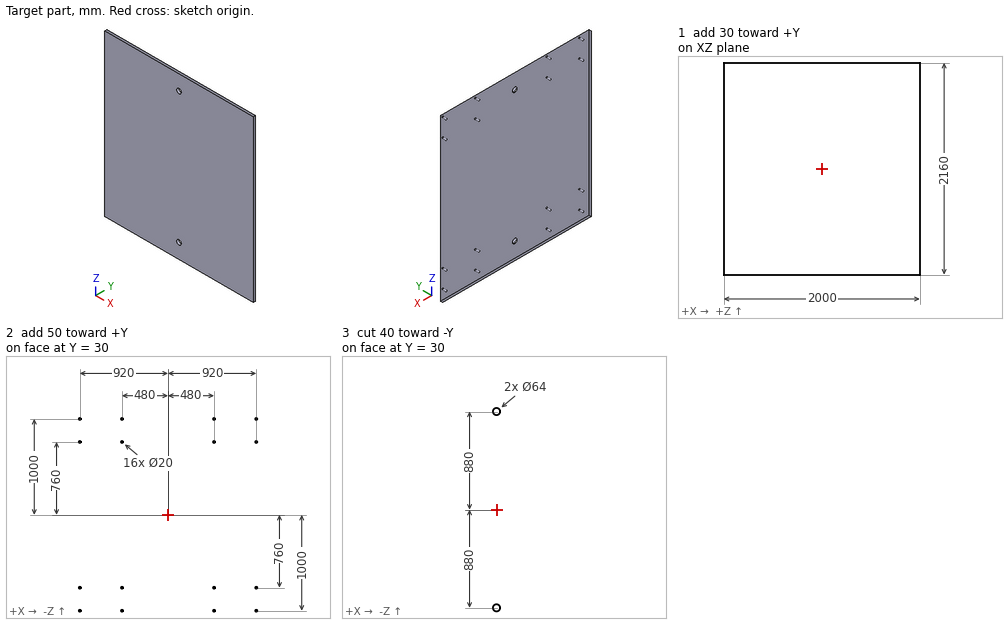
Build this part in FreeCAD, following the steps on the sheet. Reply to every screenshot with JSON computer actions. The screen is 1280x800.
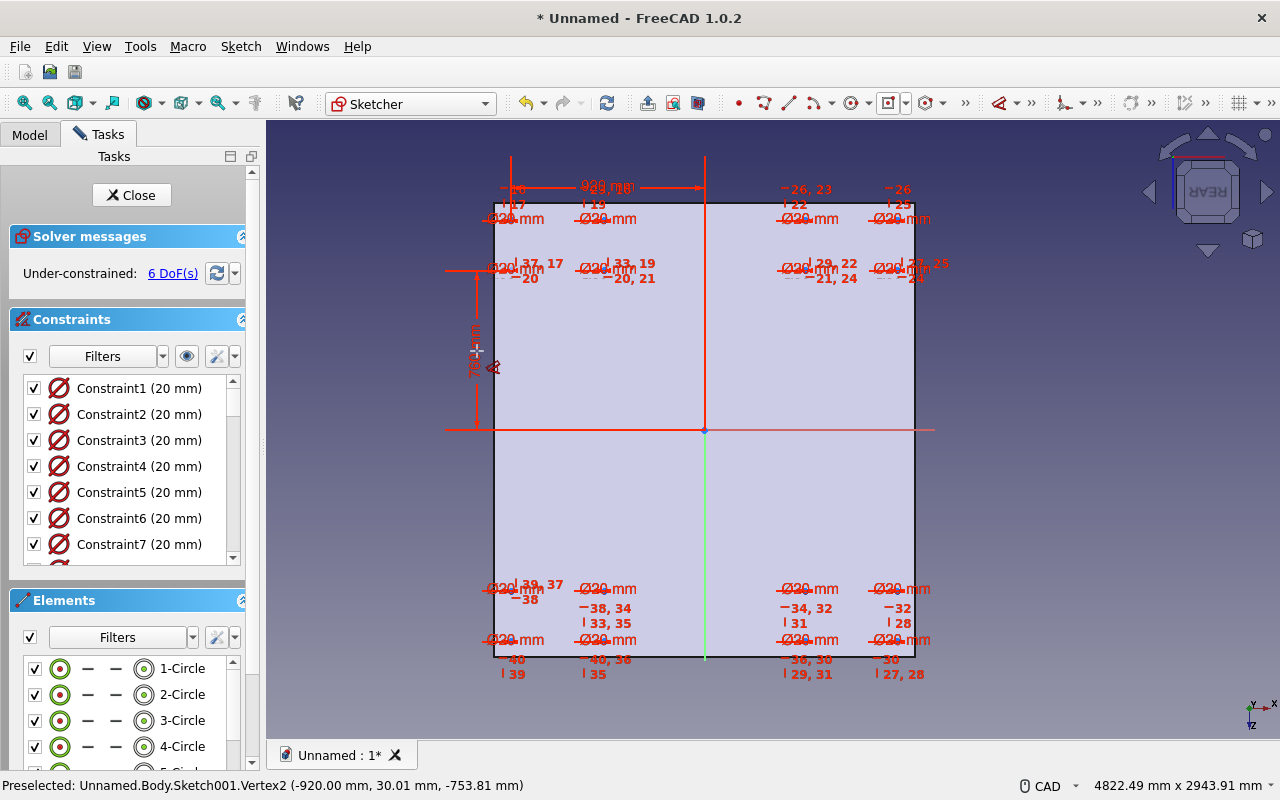
{"action": "left_click", "coordinate": [604, 221]}
{"action": "left_click", "coordinate": [690, 187]}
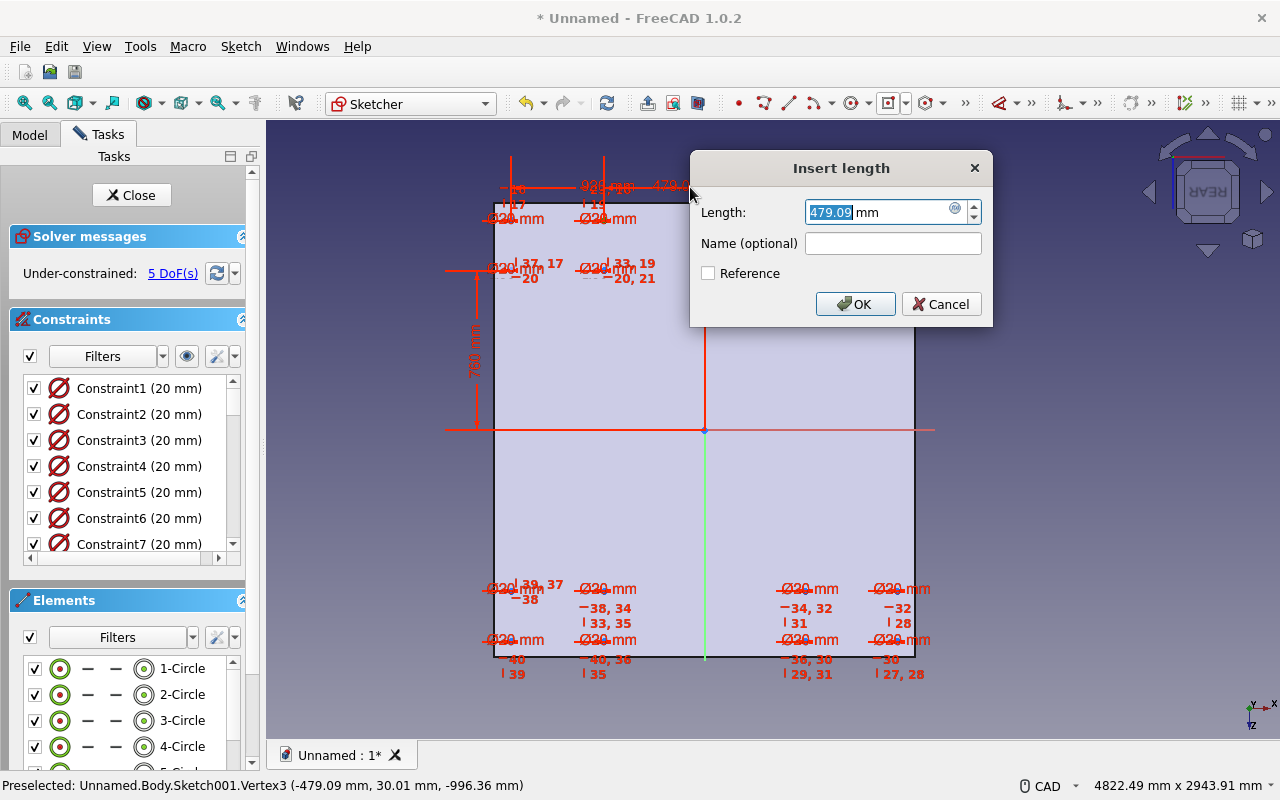
{"action": "type", "text": "480"}
{"action": "key", "text": "Return"}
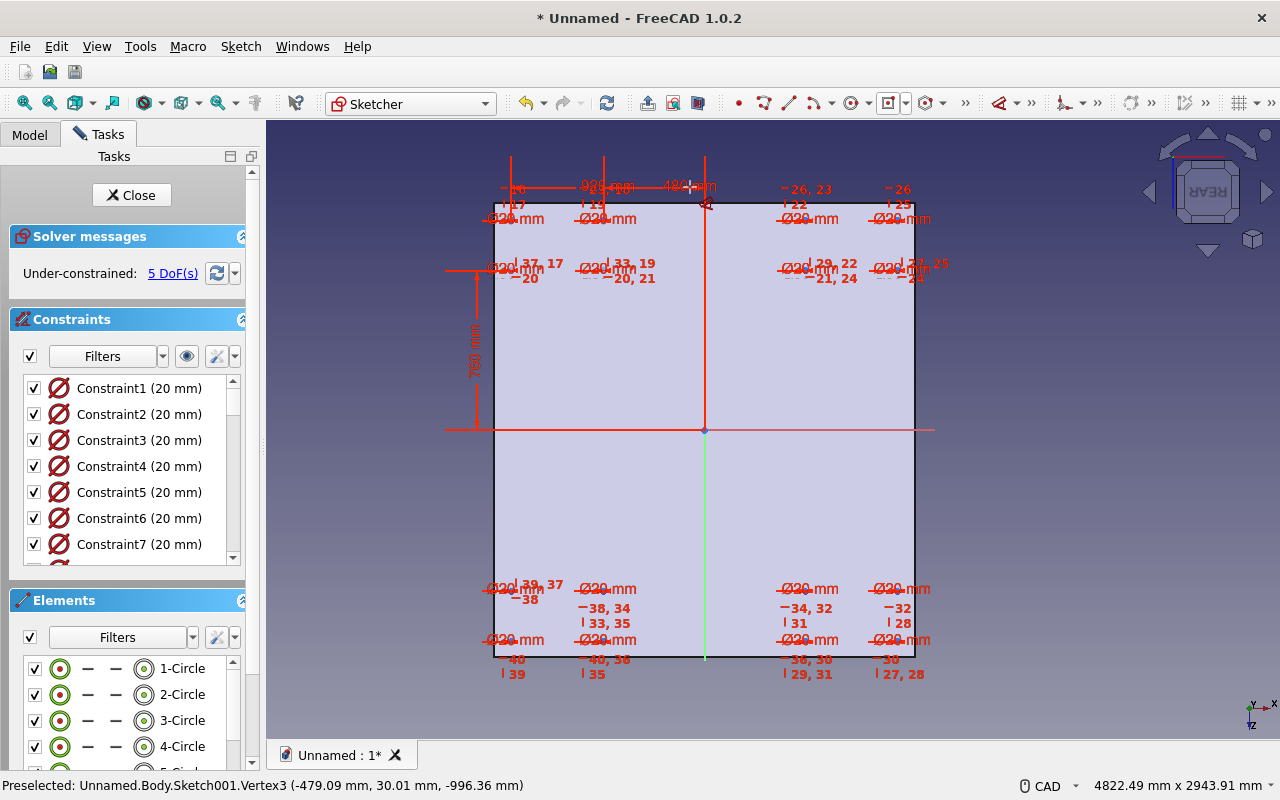
{"action": "left_click", "coordinate": [806, 271]}
{"action": "left_click", "coordinate": [755, 237]}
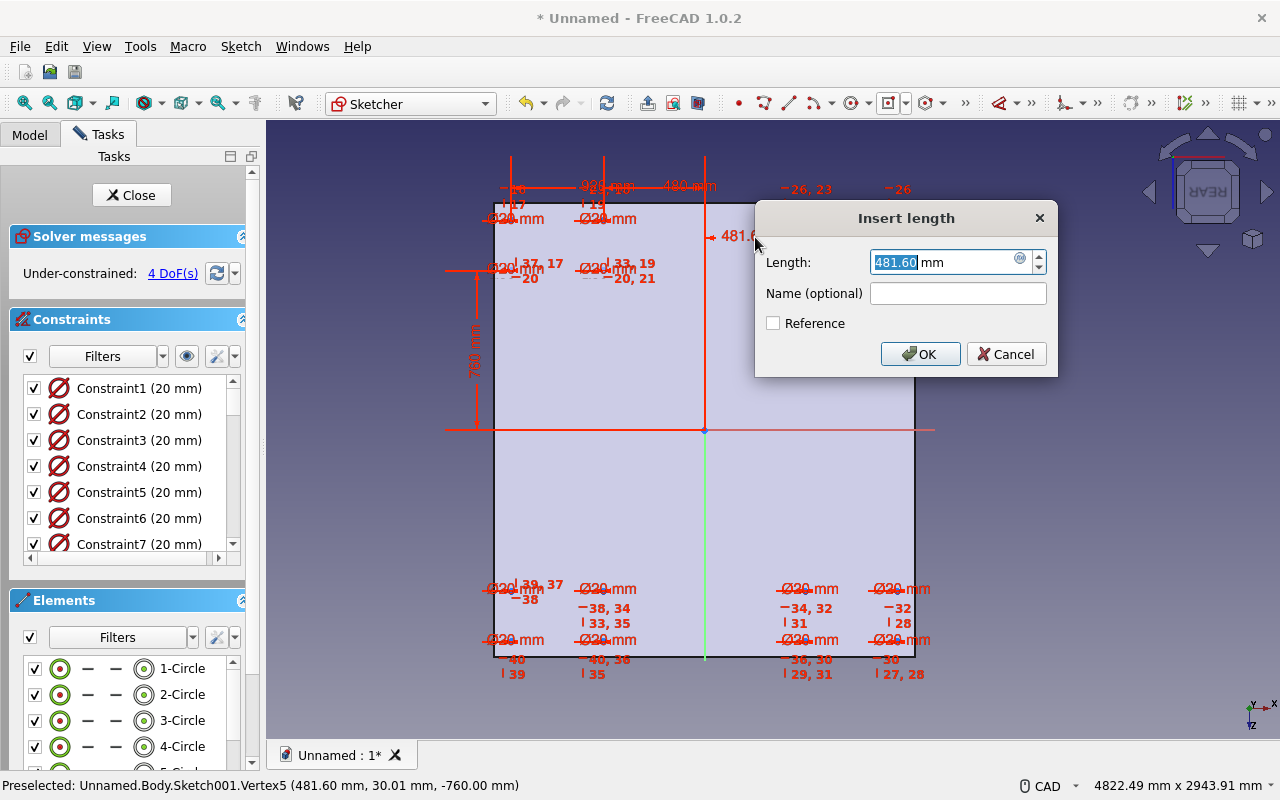
{"action": "type", "text": "480"}
{"action": "key", "text": "Return"}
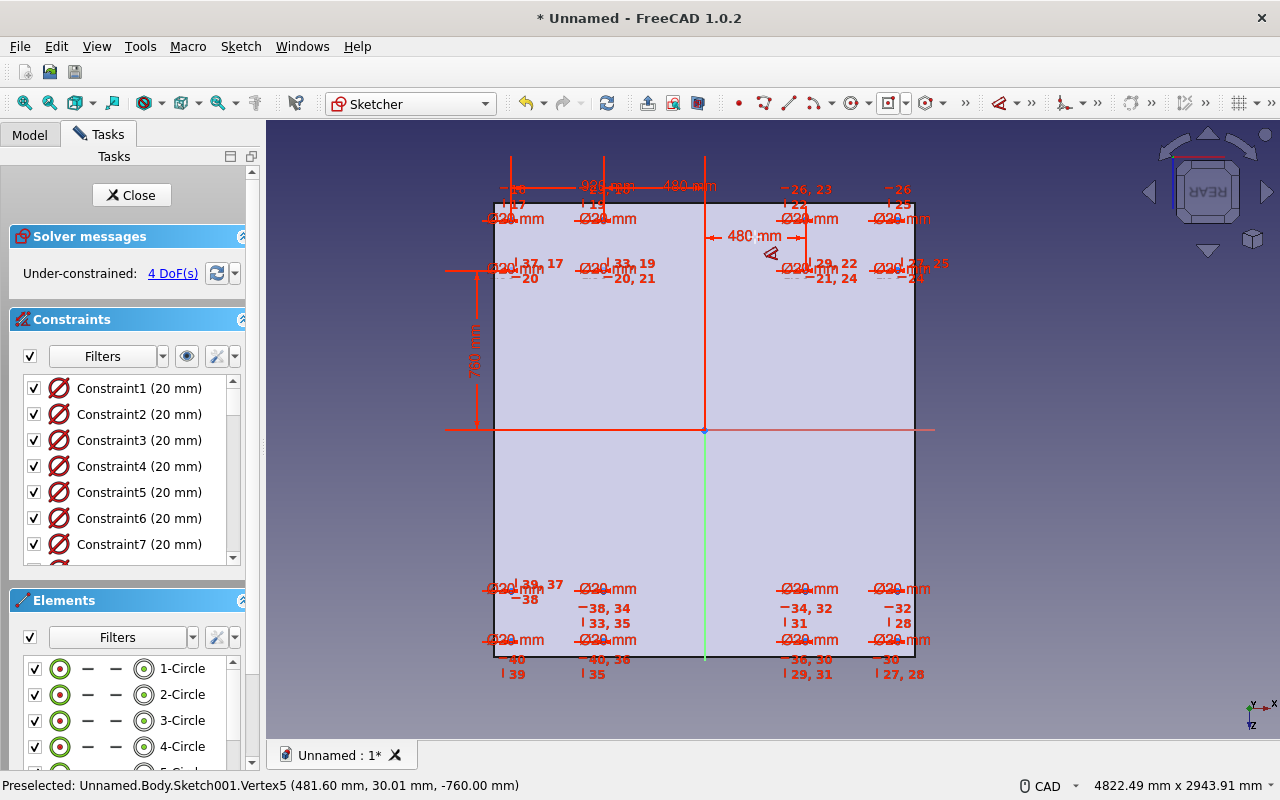
{"action": "left_click", "coordinate": [898, 271]}
{"action": "left_click", "coordinate": [846, 237]}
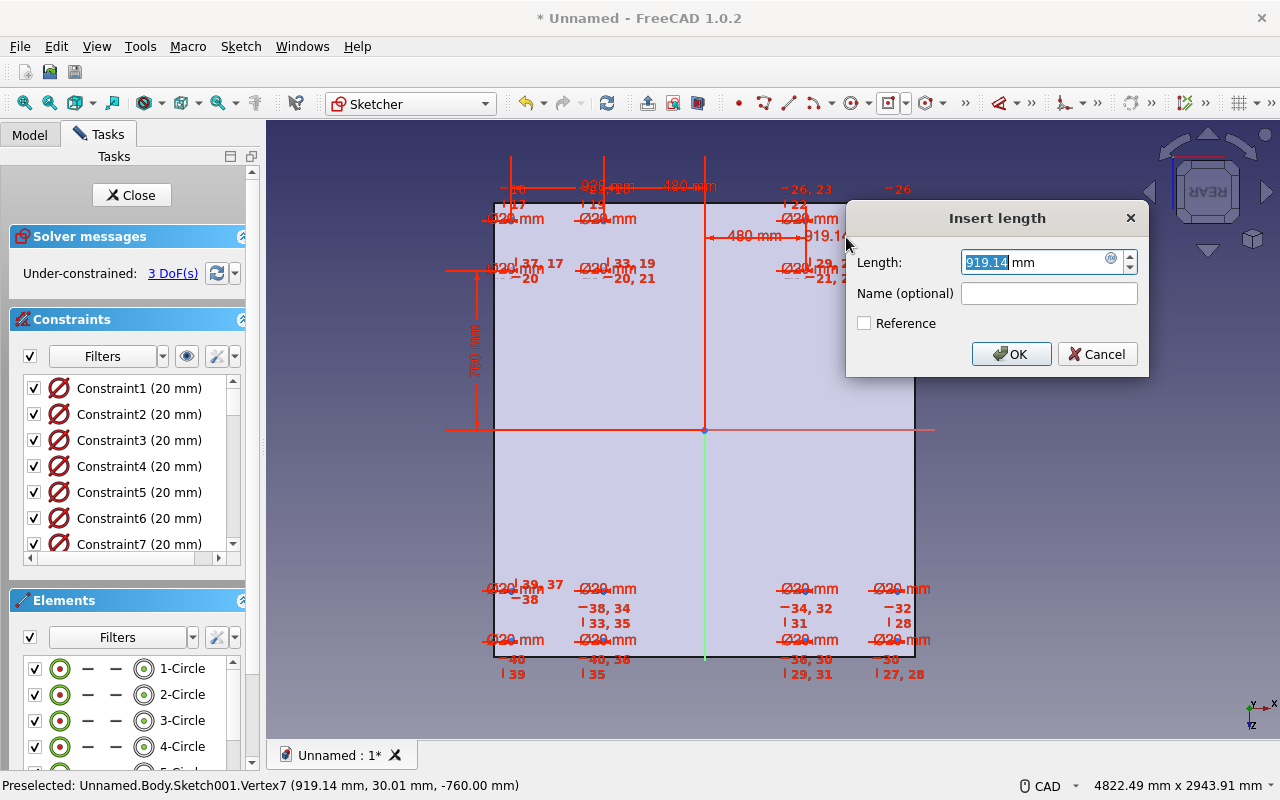
{"action": "type", "text": "920"}
{"action": "key", "text": "Return"}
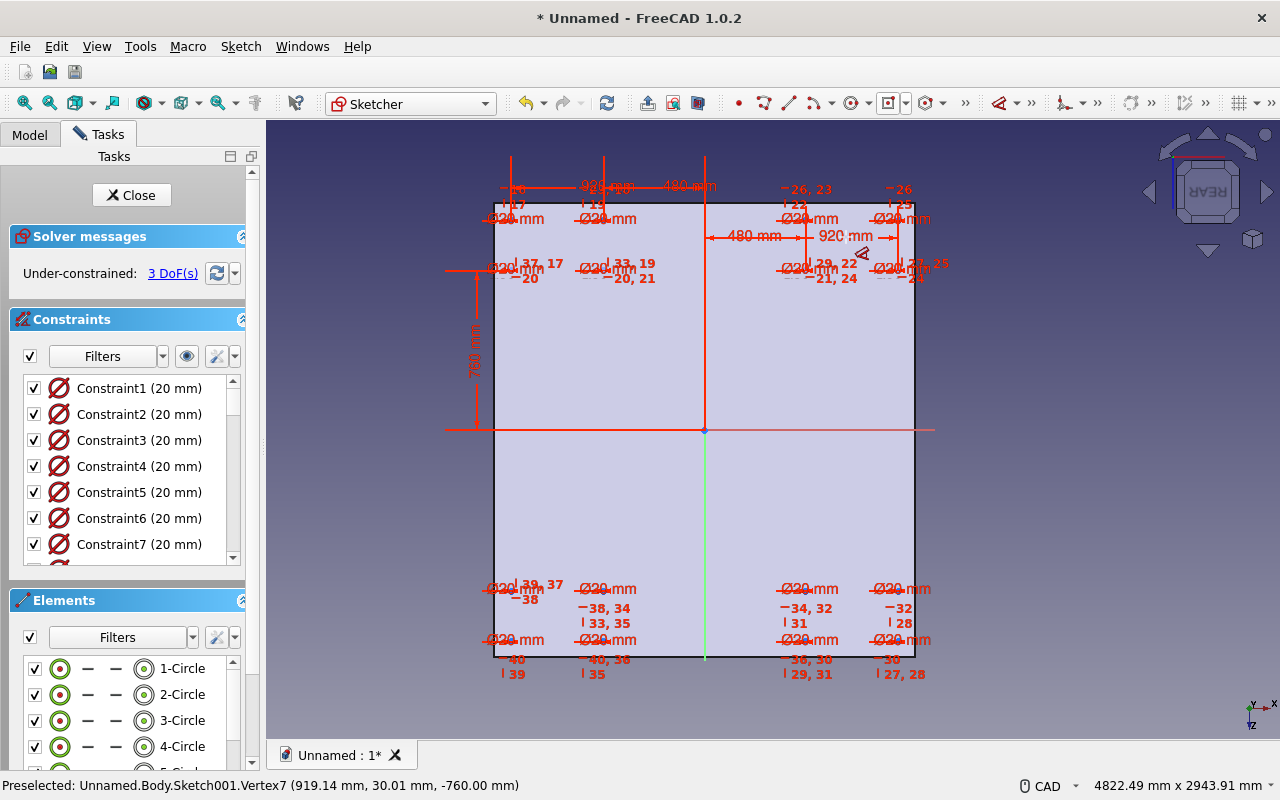
{"action": "left_click", "coordinate": [898, 591]}
{"action": "left_click", "coordinate": [932, 511]}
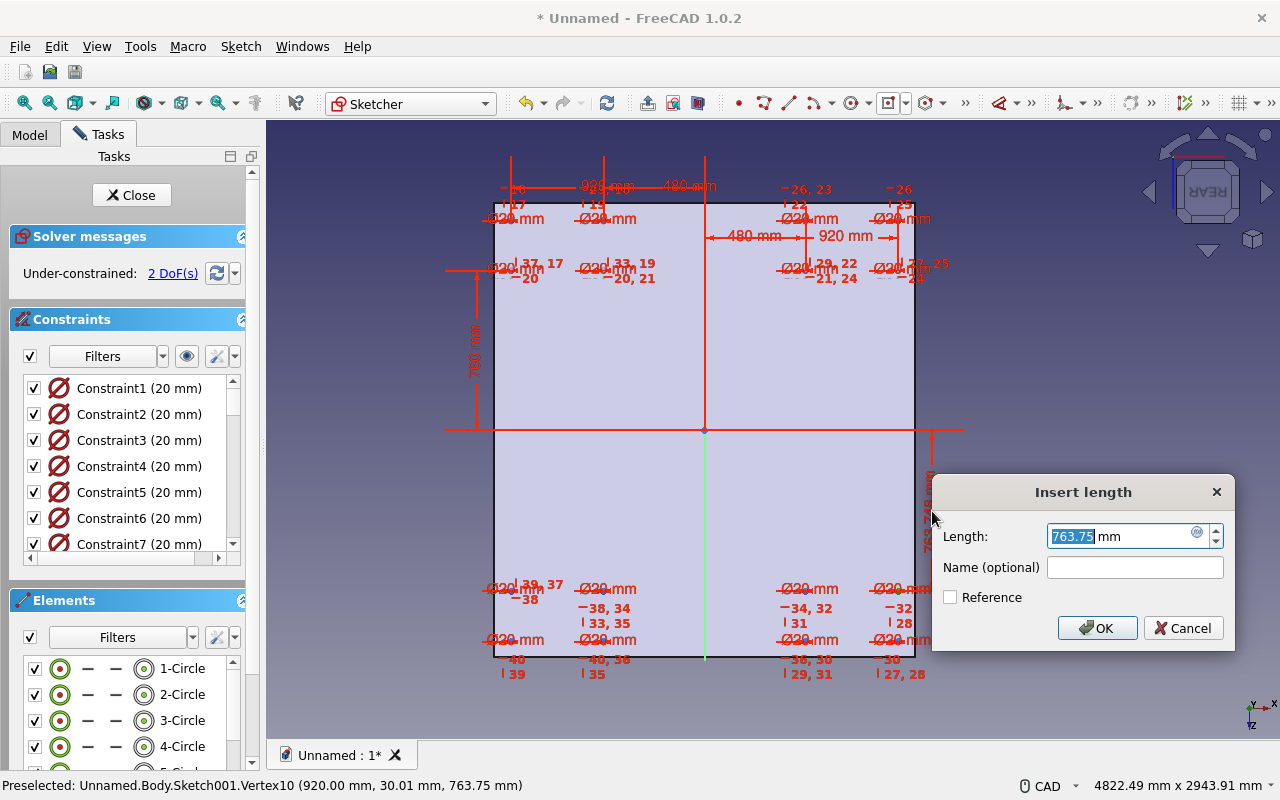
{"action": "type", "text": "760"}
{"action": "key", "text": "Return"}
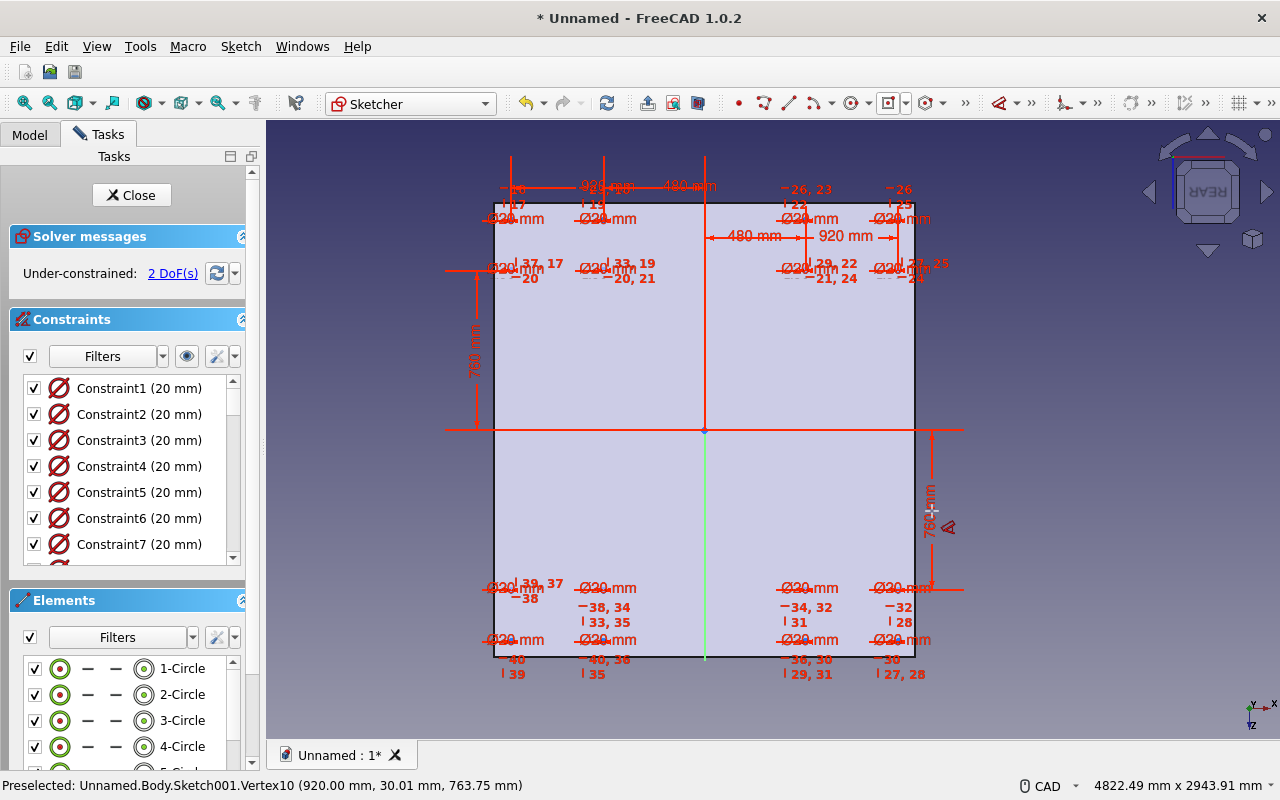
{"action": "left_click", "coordinate": [511, 221]}
{"action": "left_click", "coordinate": [477, 326]}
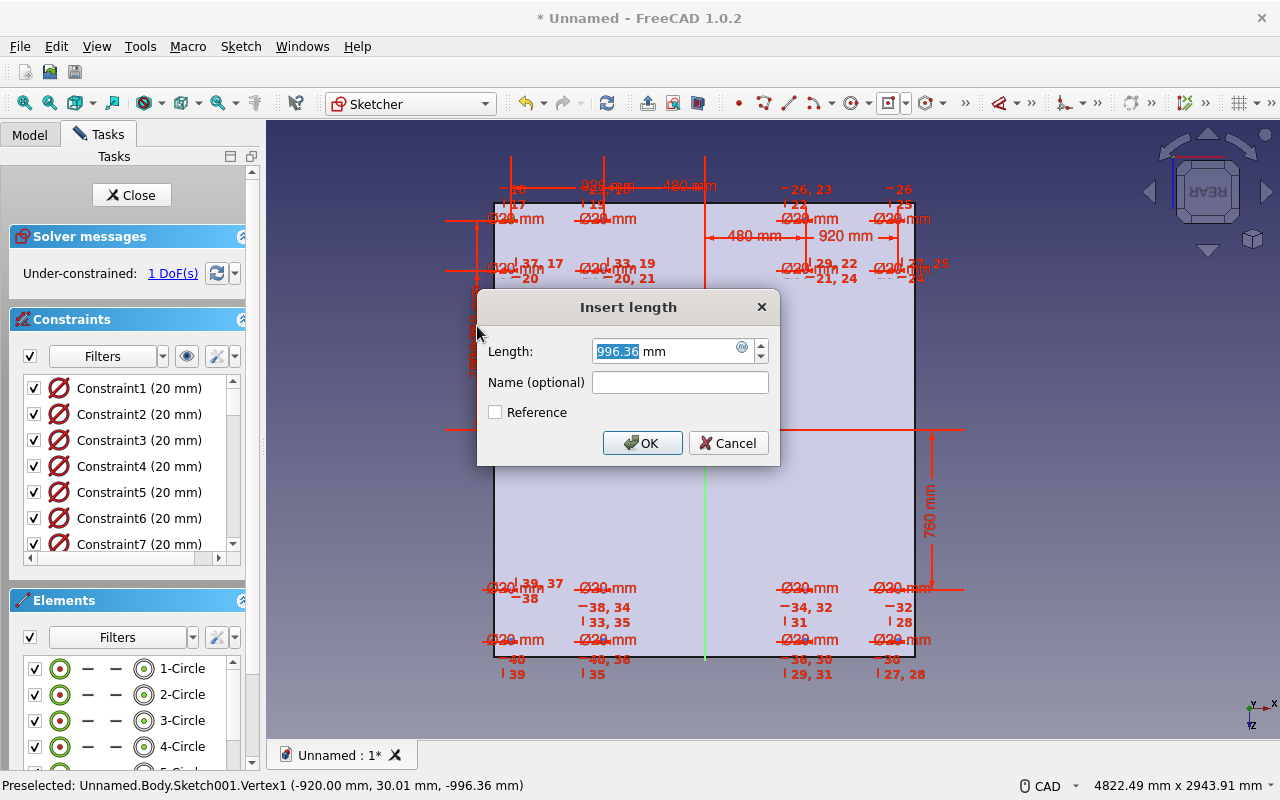
{"action": "type", "text": "1000"}
{"action": "key", "text": "Return"}